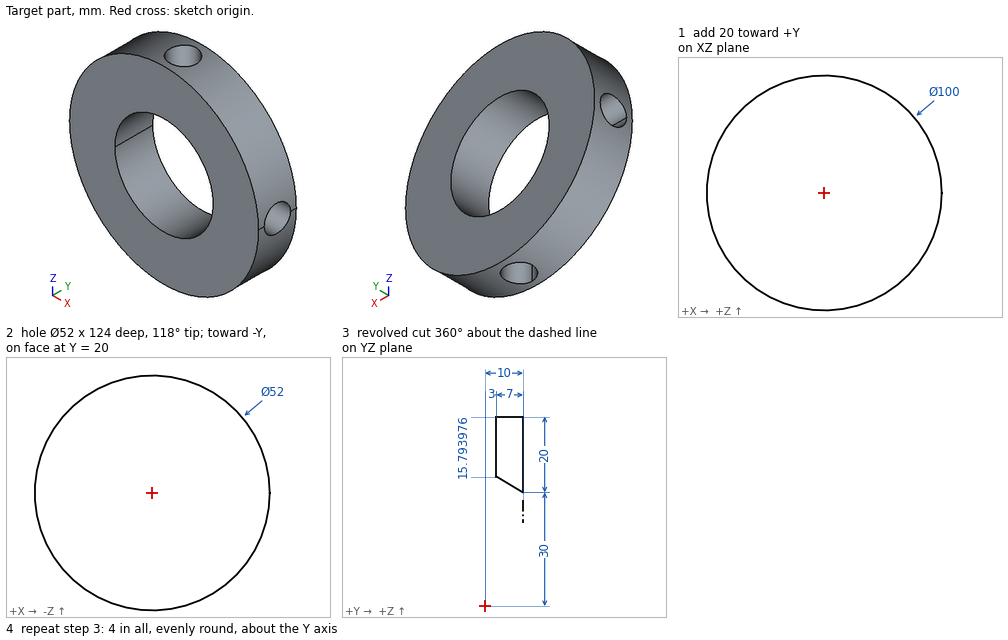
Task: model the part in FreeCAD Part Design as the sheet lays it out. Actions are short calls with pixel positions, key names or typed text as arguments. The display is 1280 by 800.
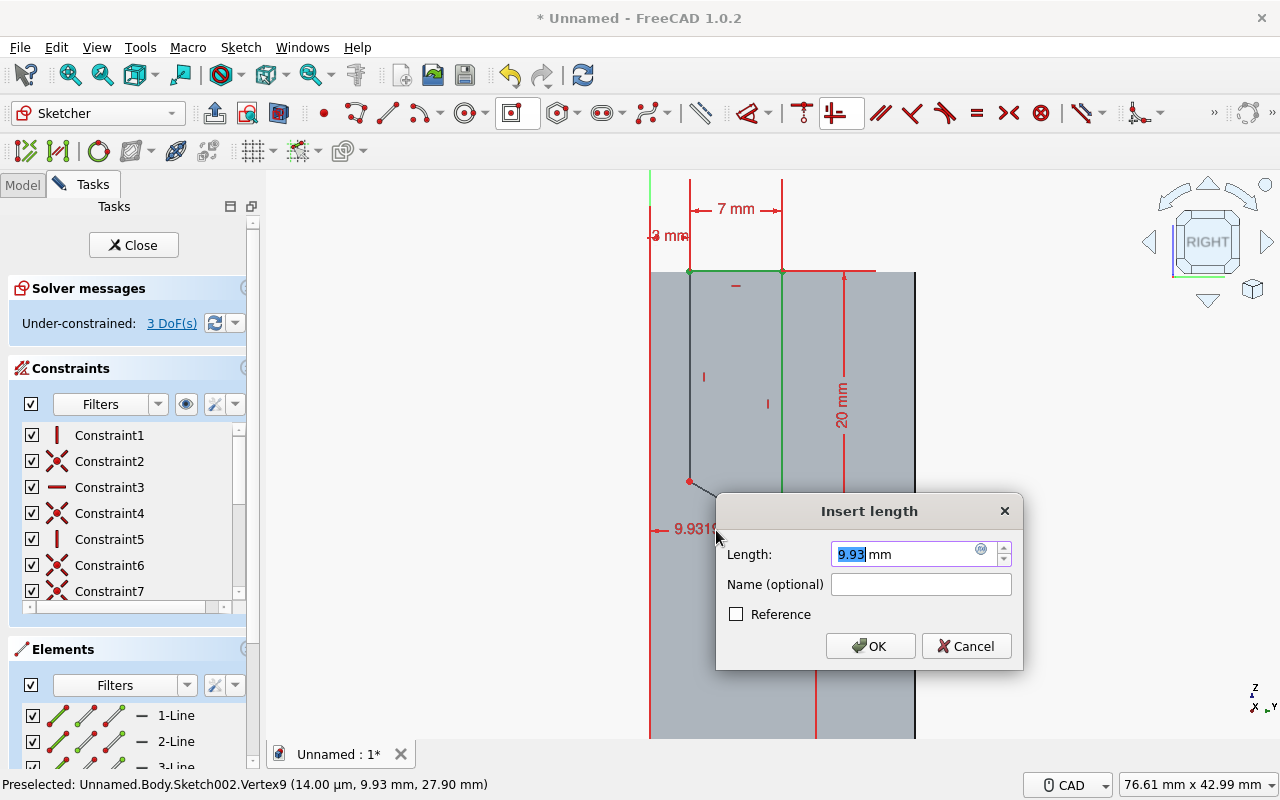
text(10)
key(Return)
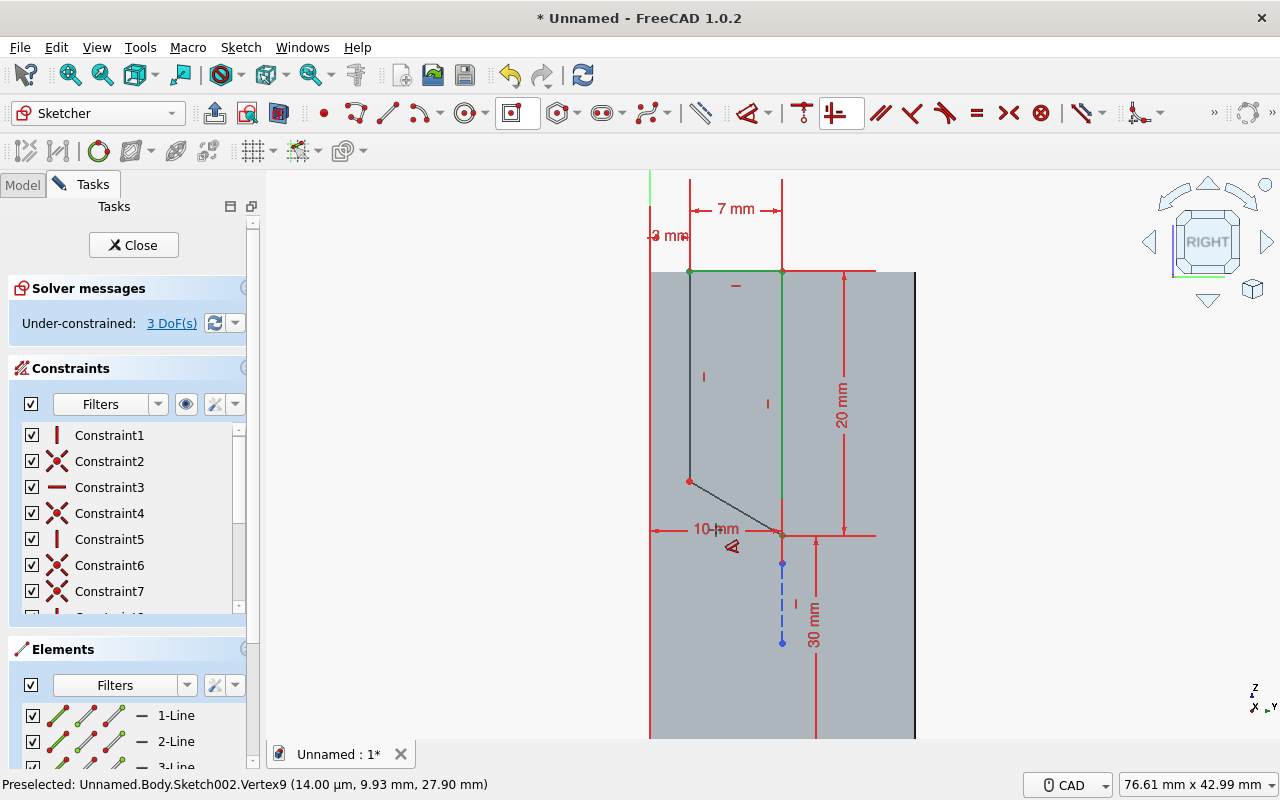
click(690, 334)
click(724, 376)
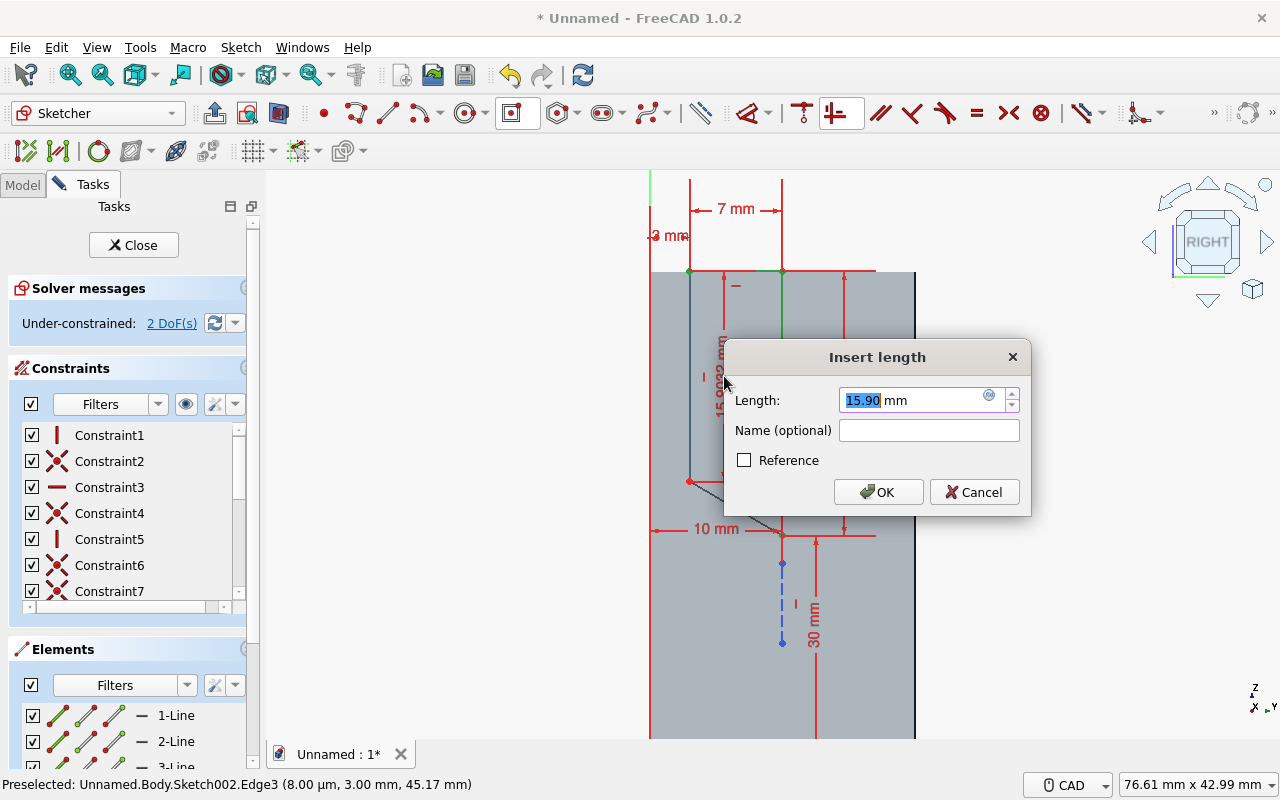
text(15.793976)
key(Return)
key(Escape)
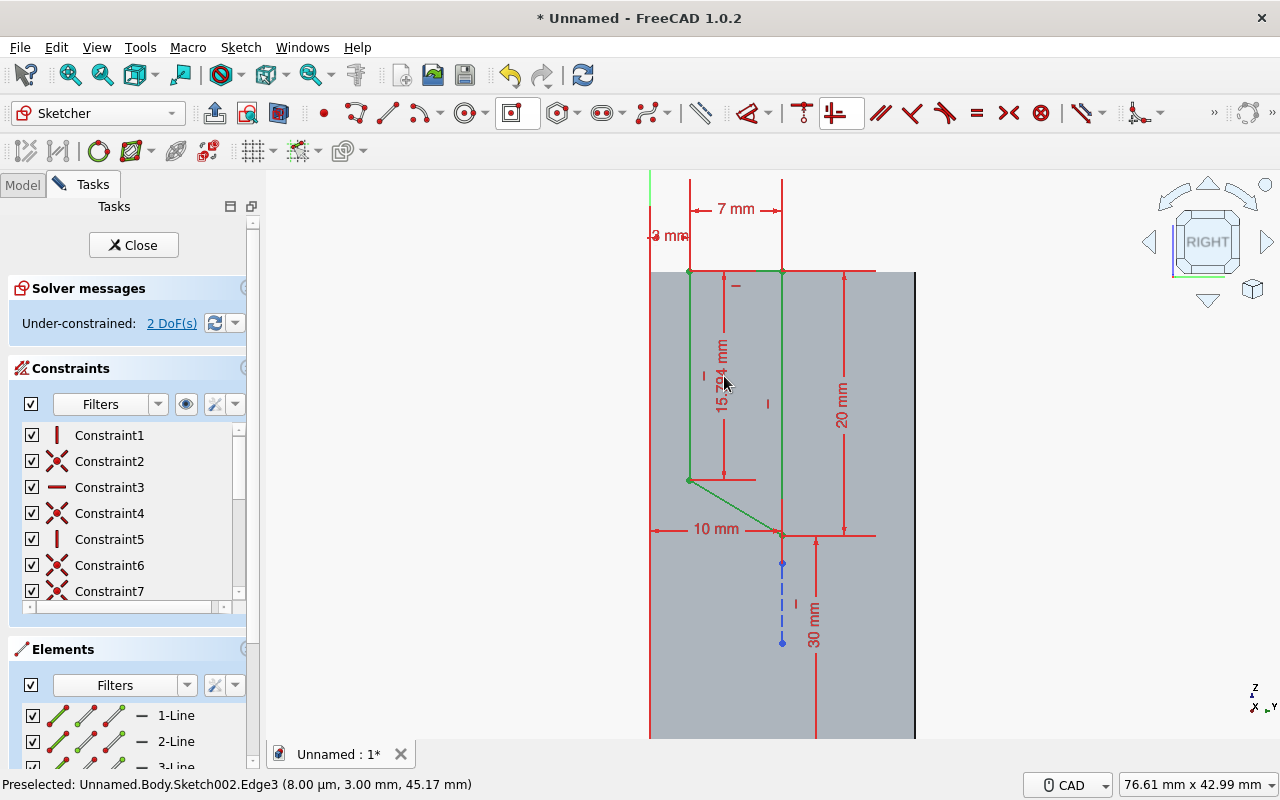
click(134, 245)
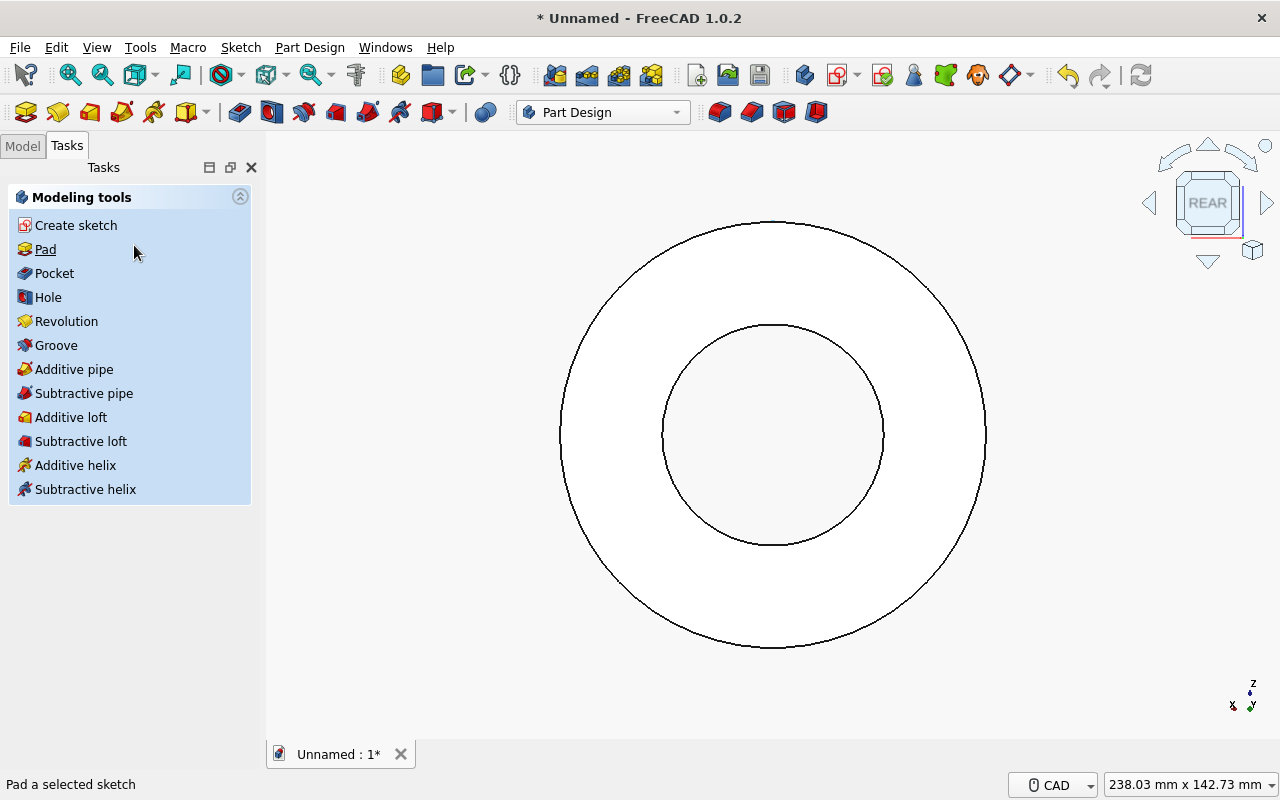
click(304, 112)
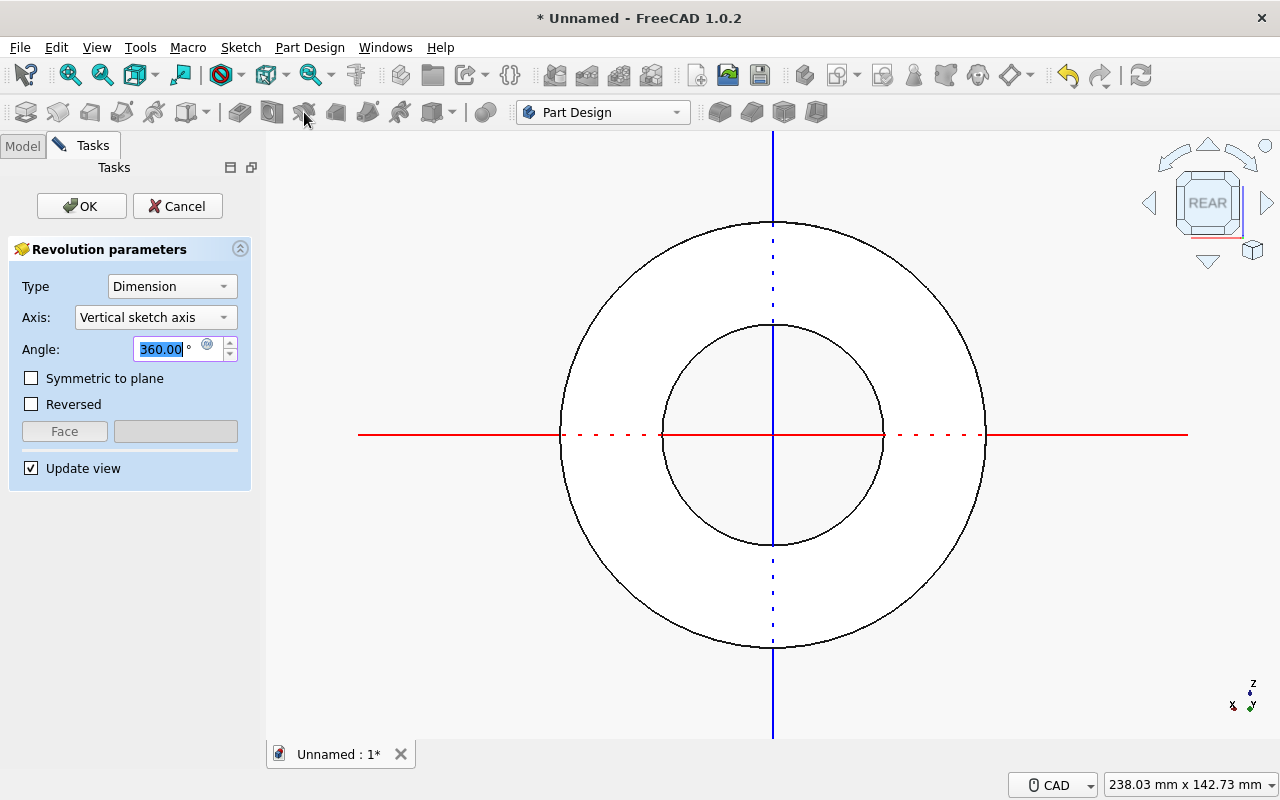
click(156, 318)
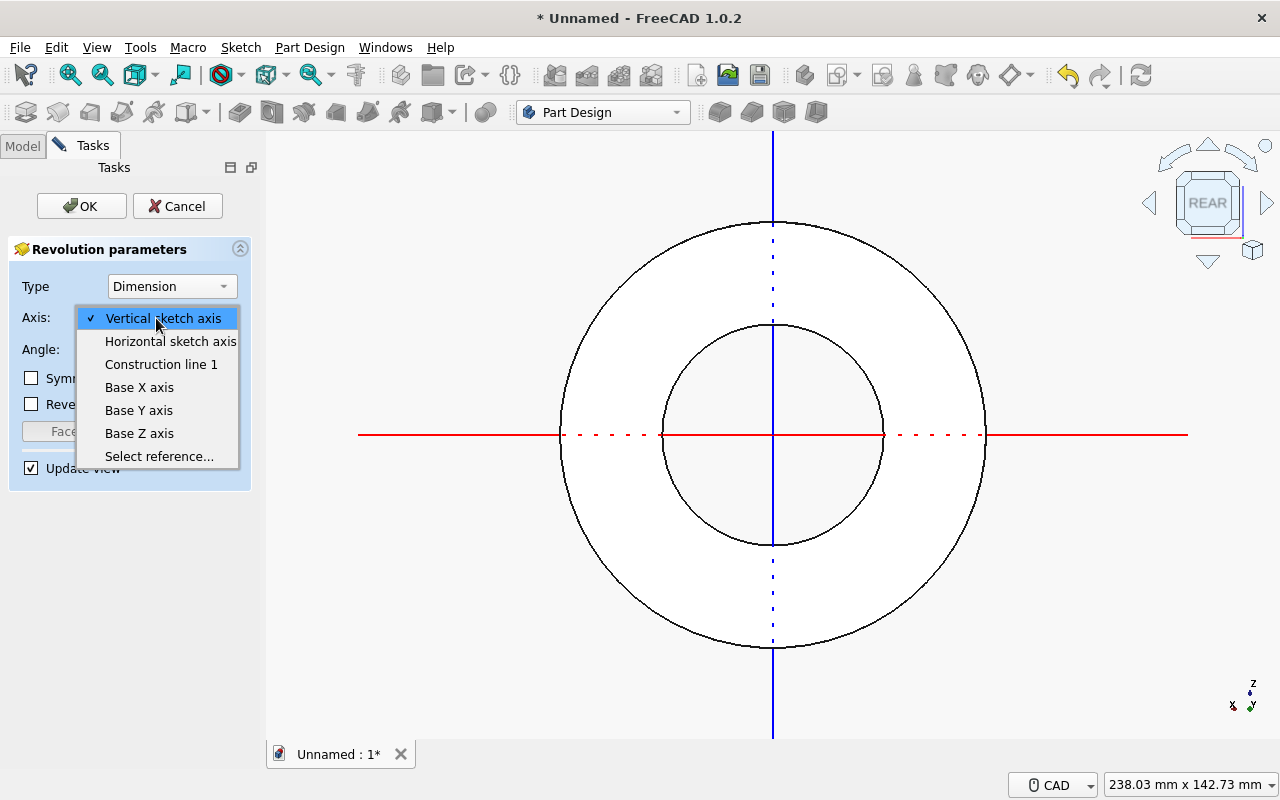
click(156, 364)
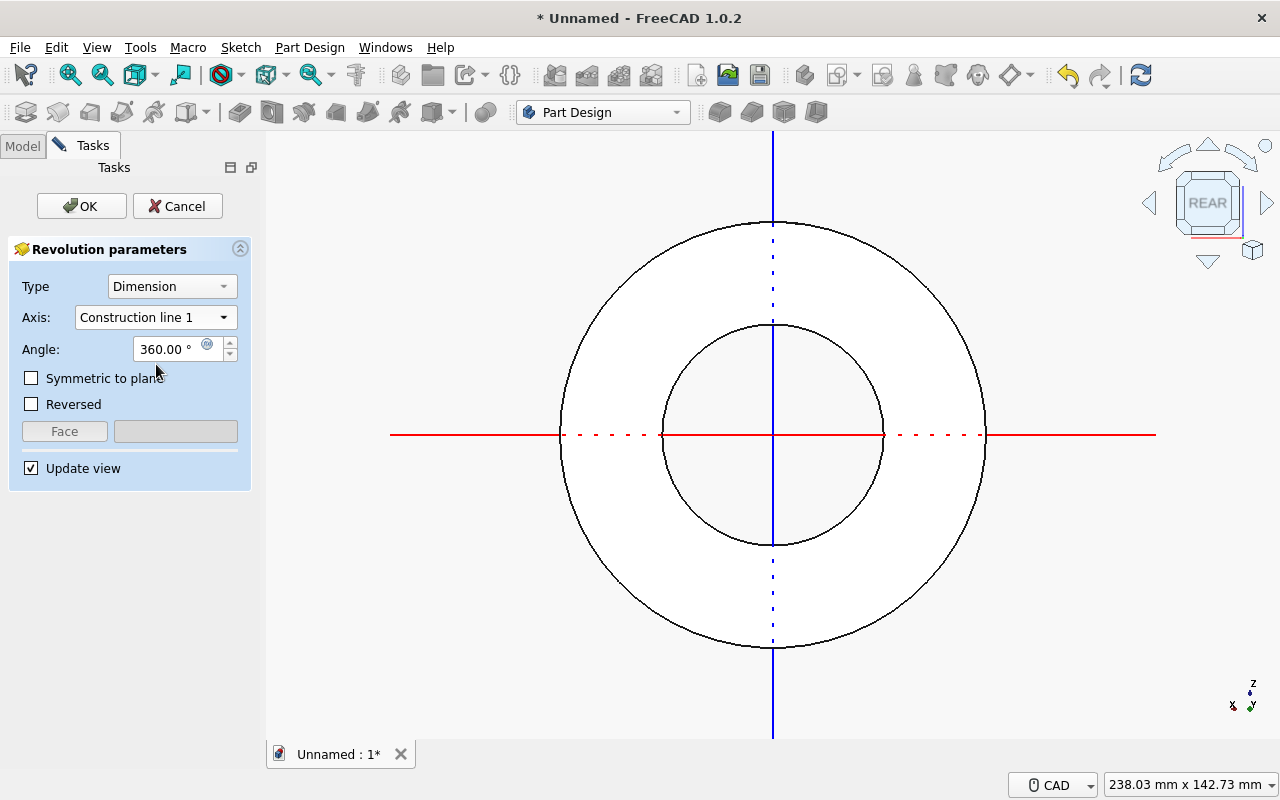
click(82, 206)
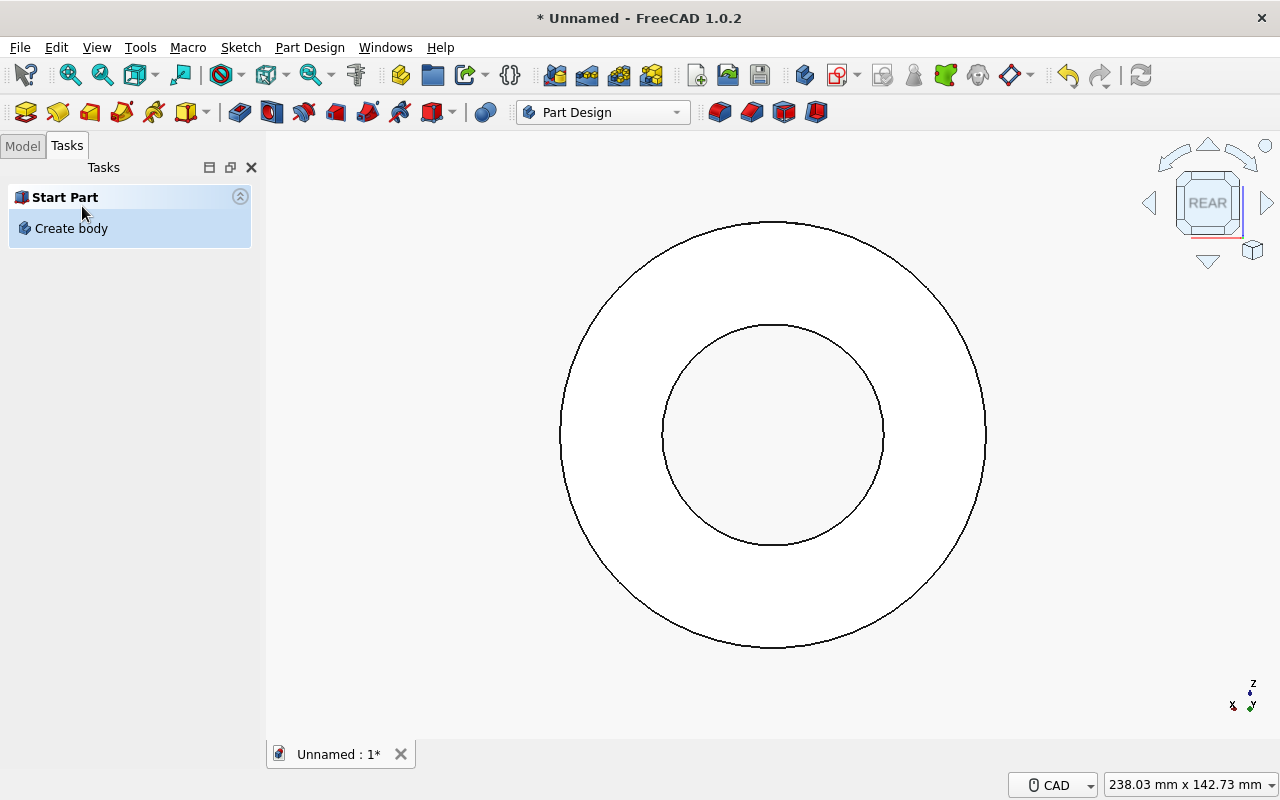
click(23, 145)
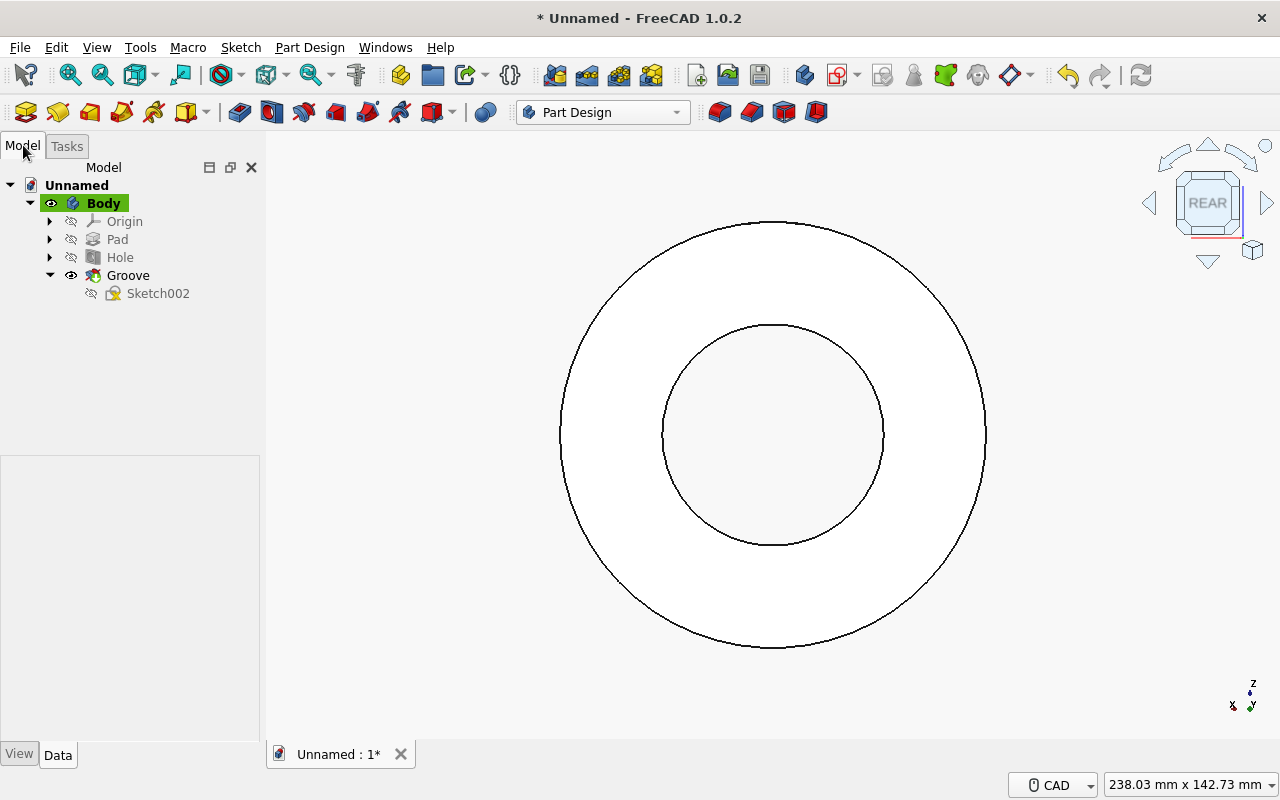
click(116, 275)